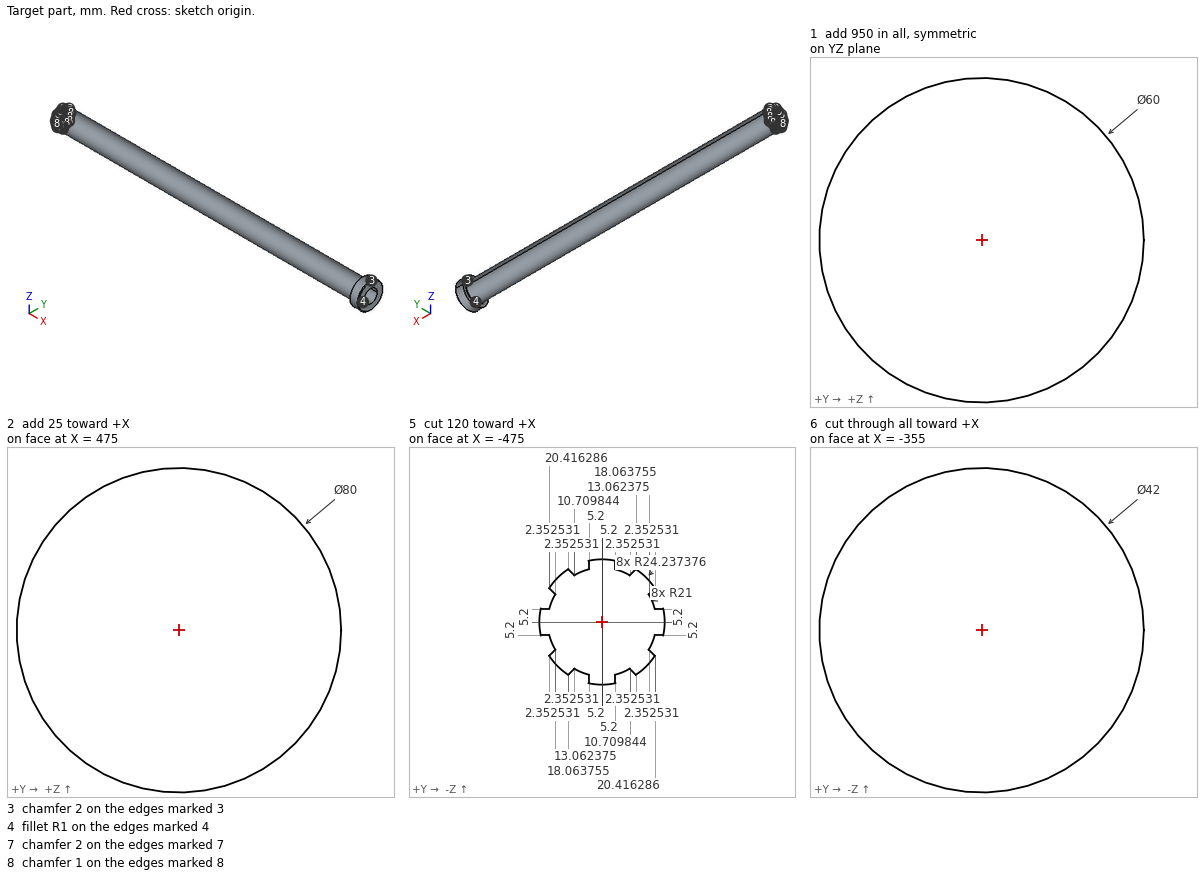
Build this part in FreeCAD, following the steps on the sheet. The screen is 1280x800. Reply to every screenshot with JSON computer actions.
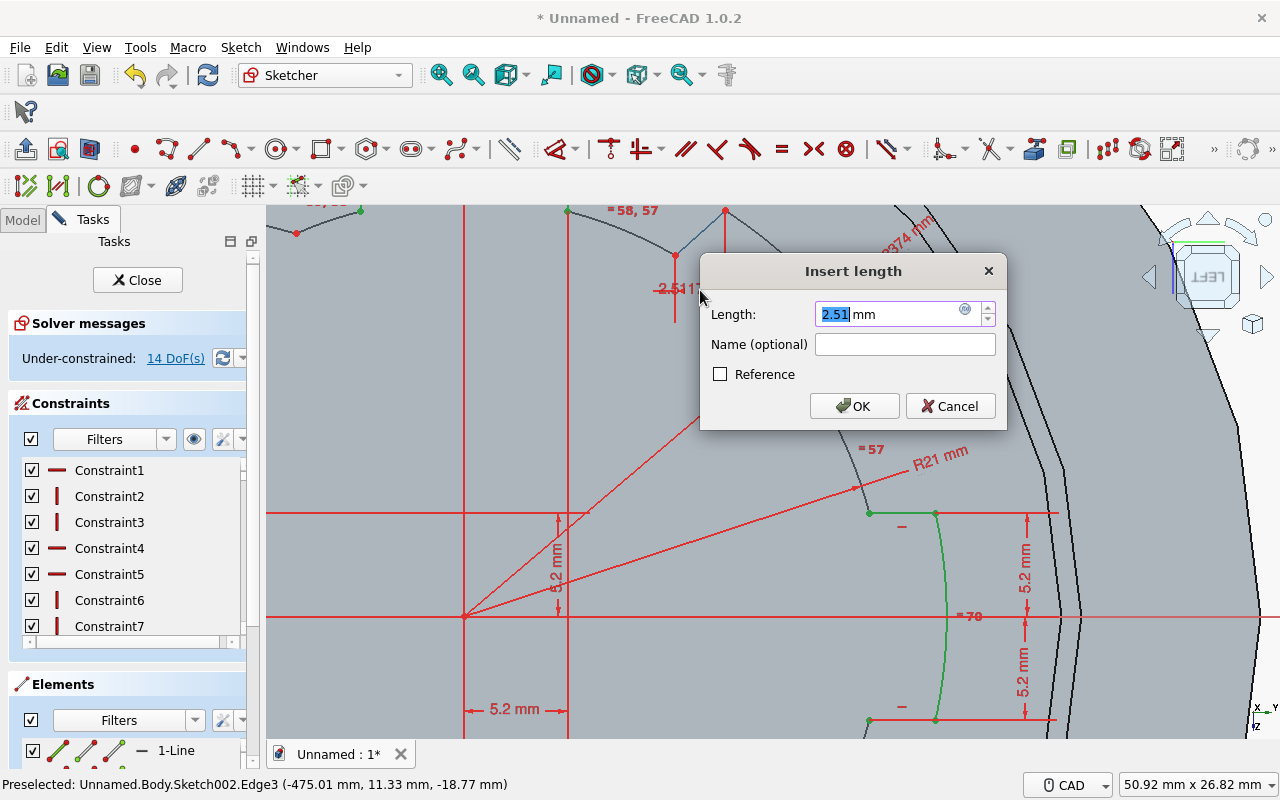
{"action": "type", "text": "2.352531"}
{"action": "key", "text": "Return"}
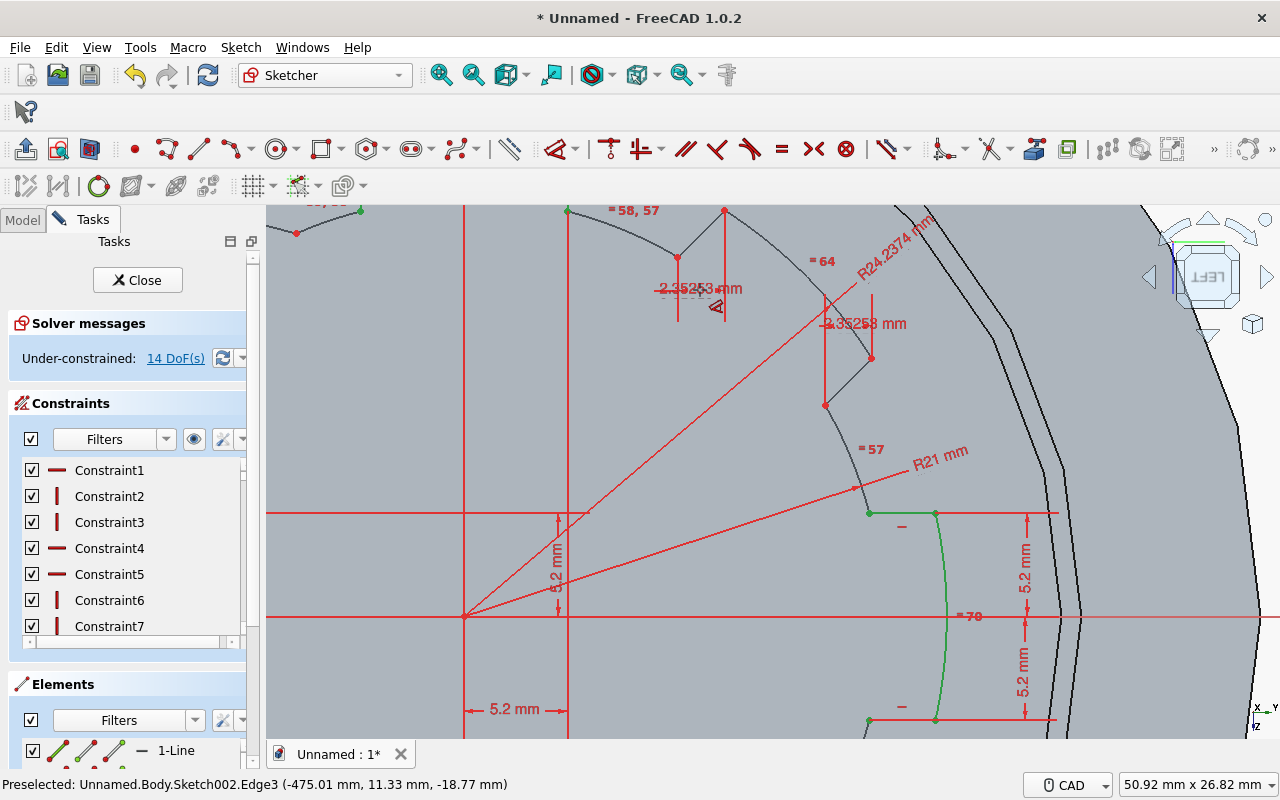
{"action": "scroll", "coordinate": [844, 388], "scroll_direction": "down", "scroll_amount": 5}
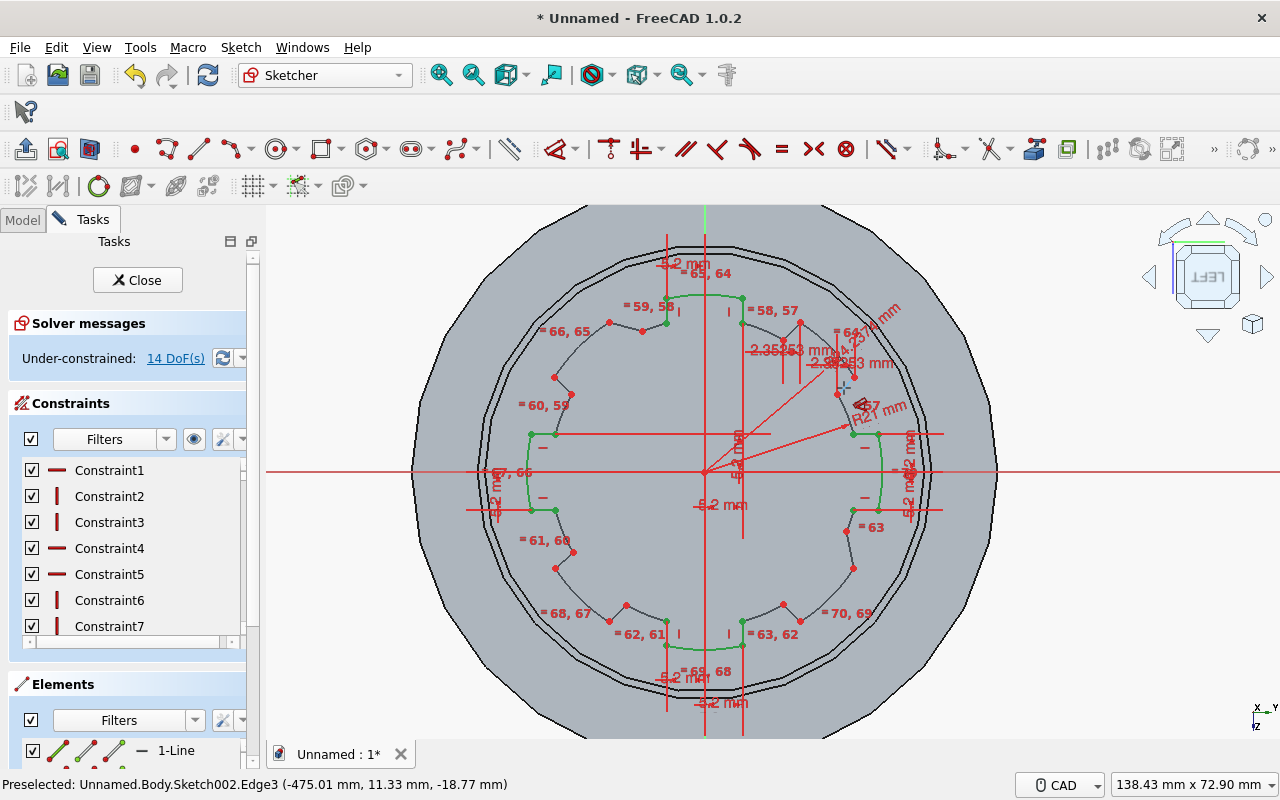
{"action": "scroll", "coordinate": [633, 329], "scroll_direction": "up", "scroll_amount": 5}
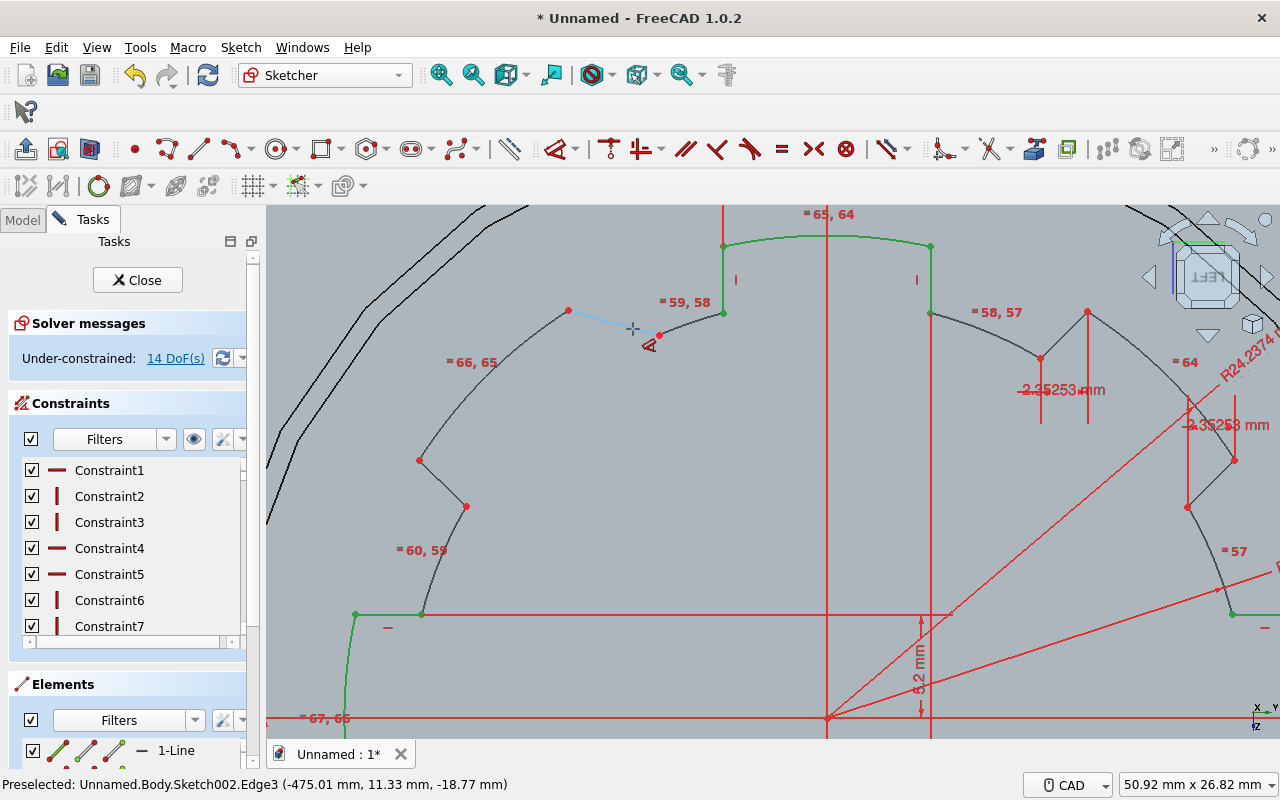
{"action": "left_click", "coordinate": [632, 328]}
{"action": "left_click", "coordinate": [614, 277]}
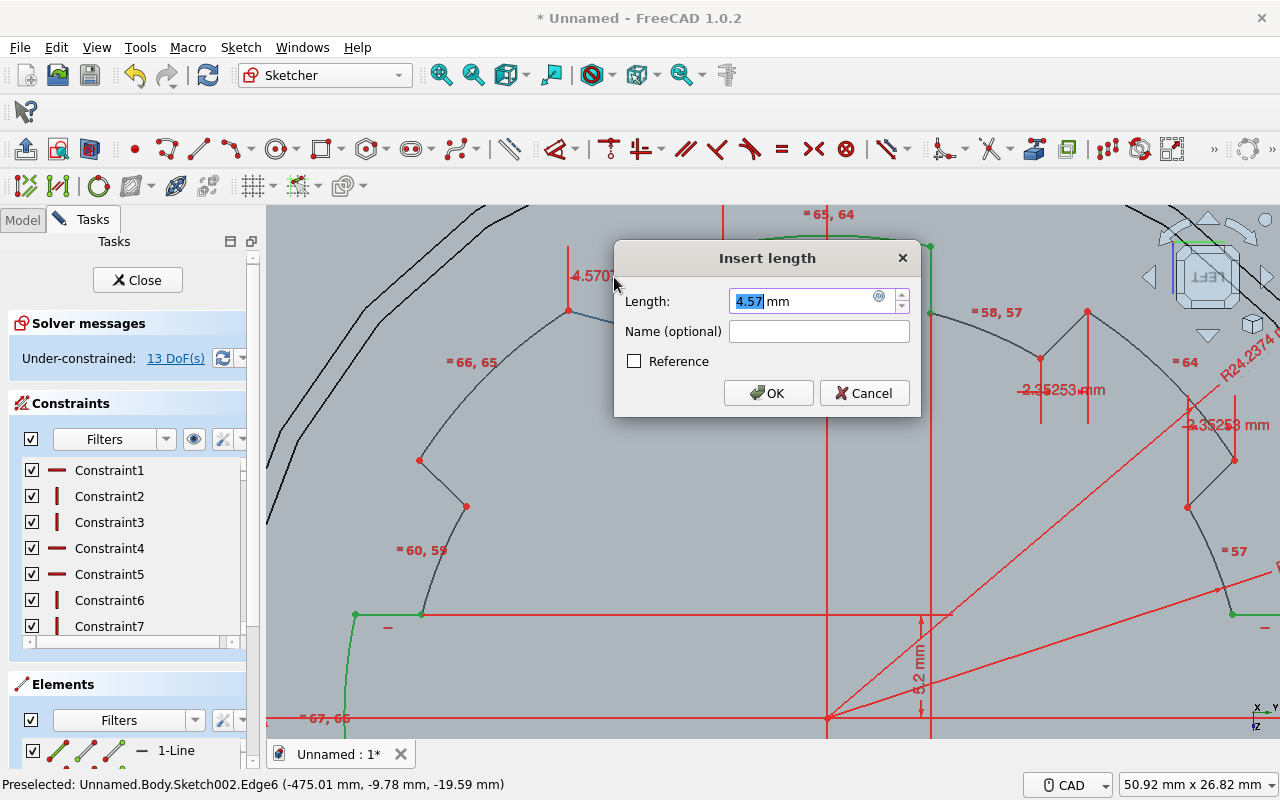
{"action": "type", "text": "2.352531"}
{"action": "key", "text": "Return"}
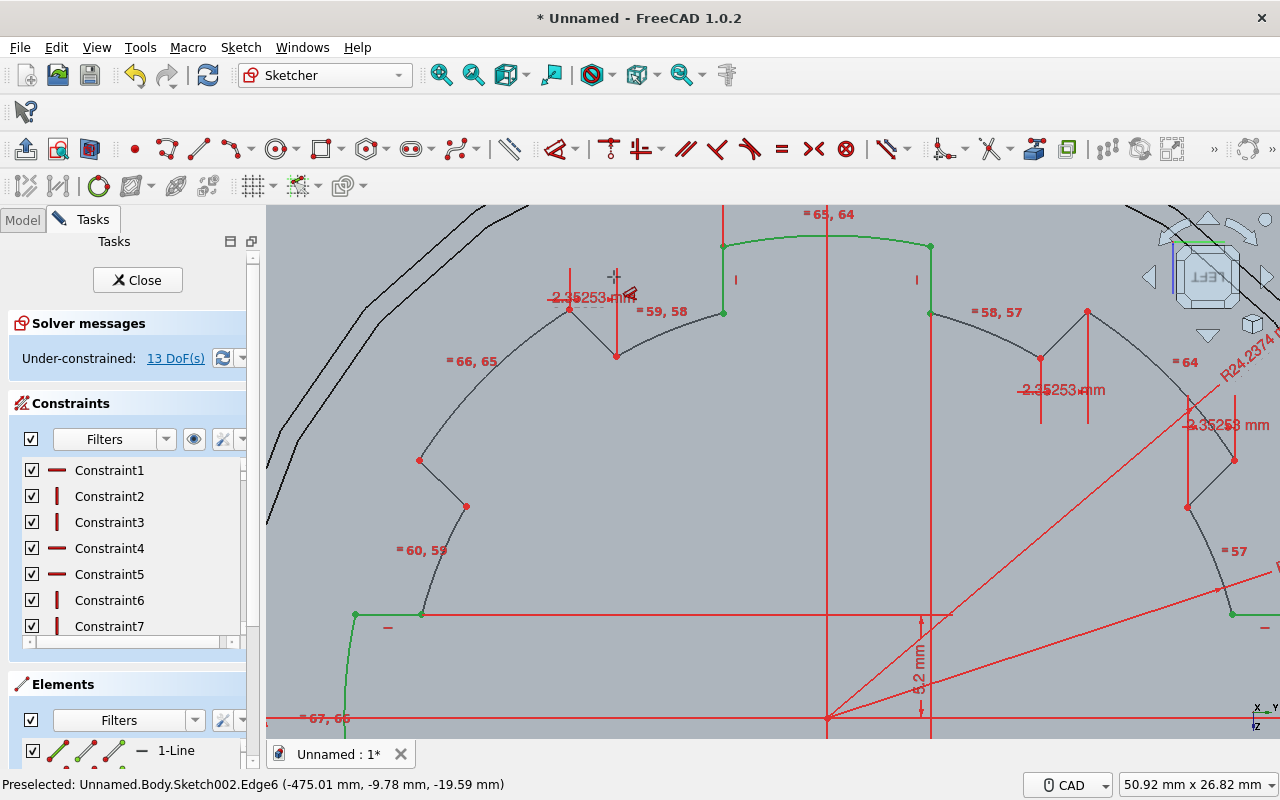
{"action": "left_click", "coordinate": [433, 474]}
{"action": "left_click", "coordinate": [426, 426]}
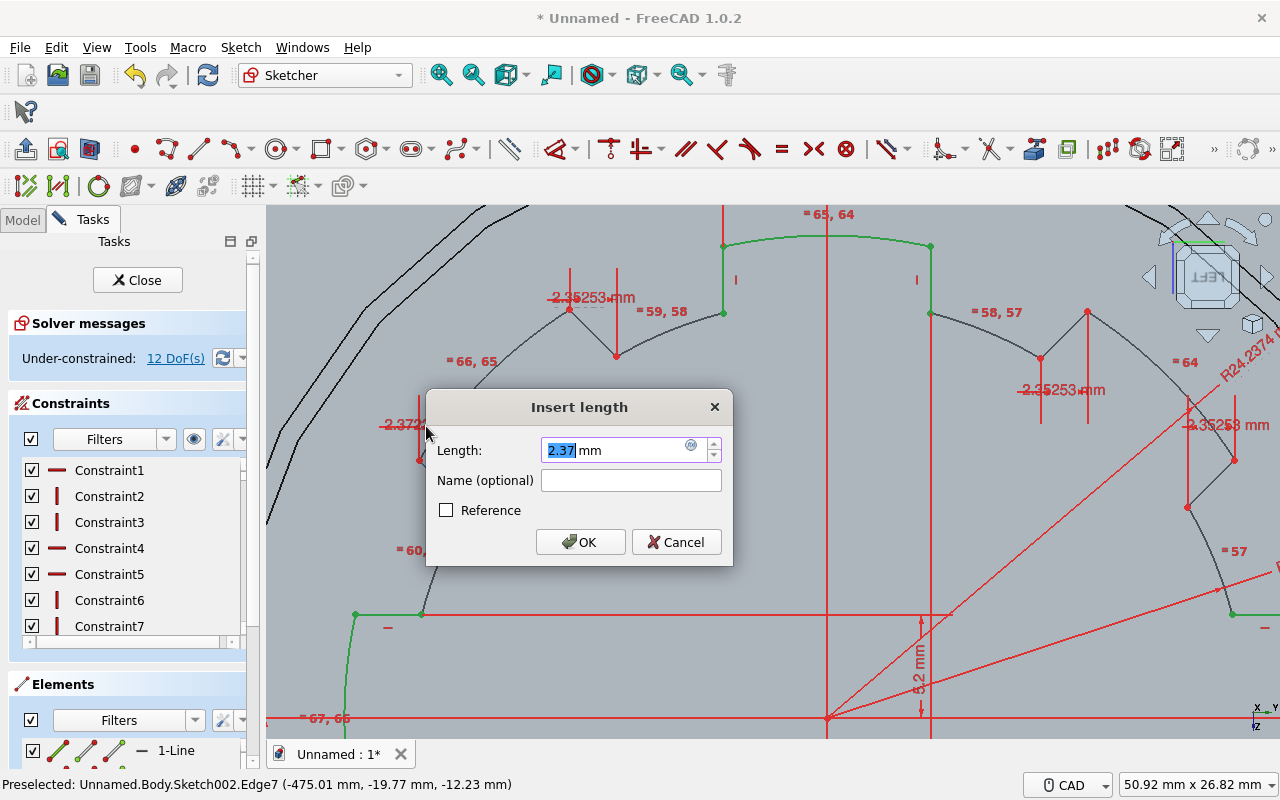
{"action": "type", "text": "2.352531"}
{"action": "key", "text": "Return"}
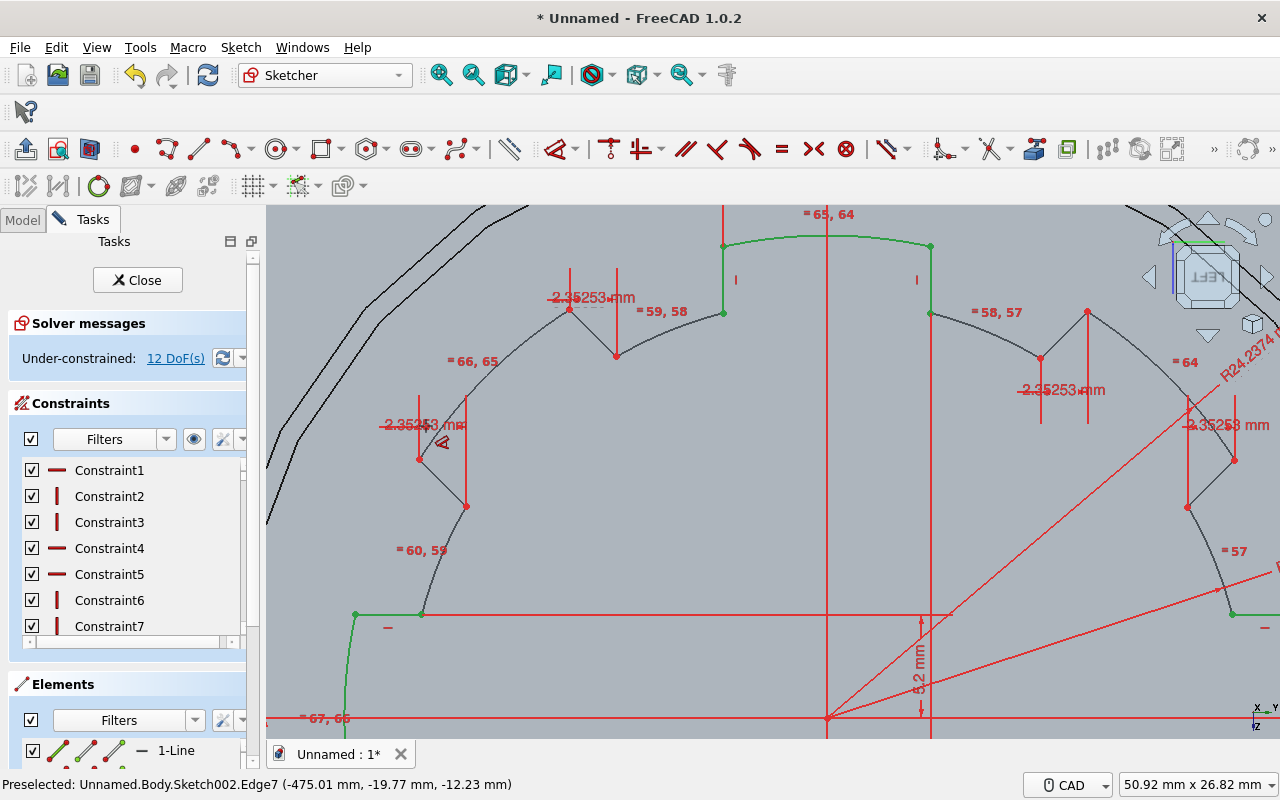
{"action": "scroll", "coordinate": [633, 329], "scroll_direction": "down", "scroll_amount": 5}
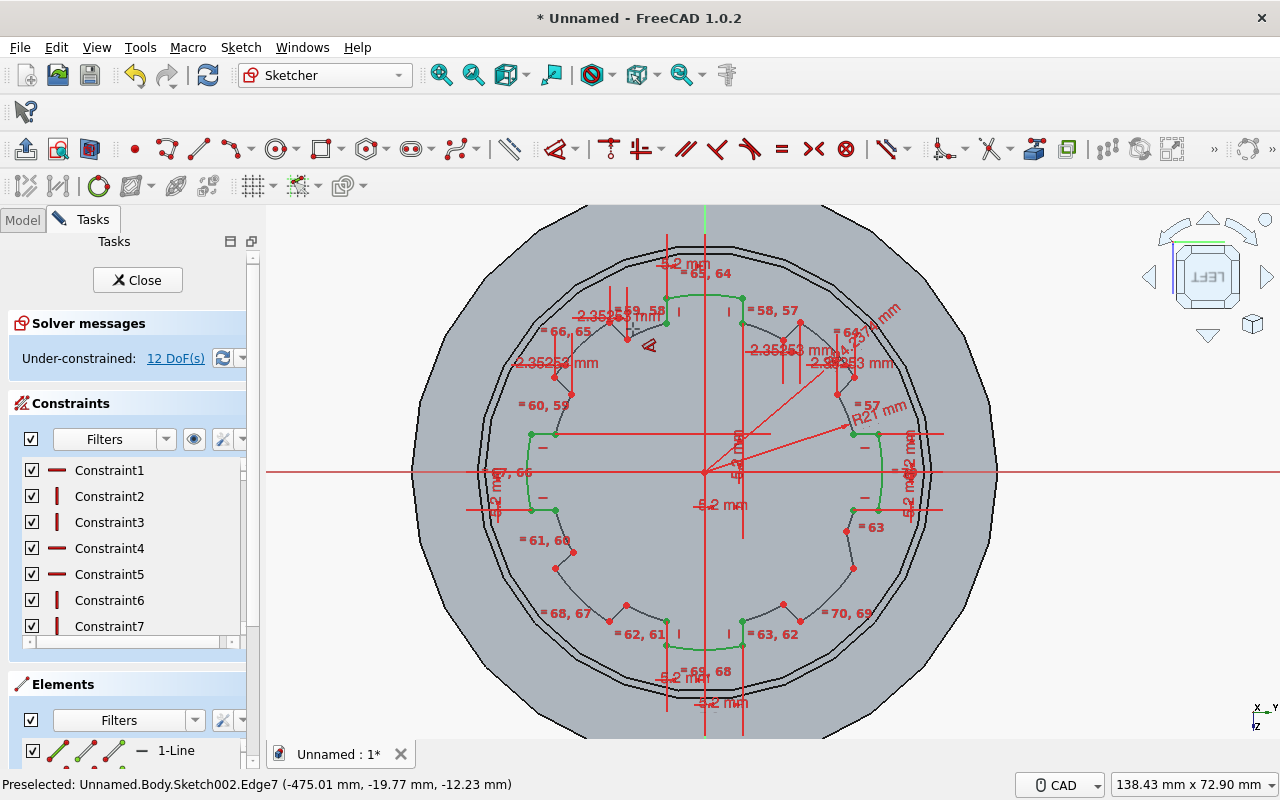
{"action": "scroll", "coordinate": [568, 557], "scroll_direction": "up", "scroll_amount": 5}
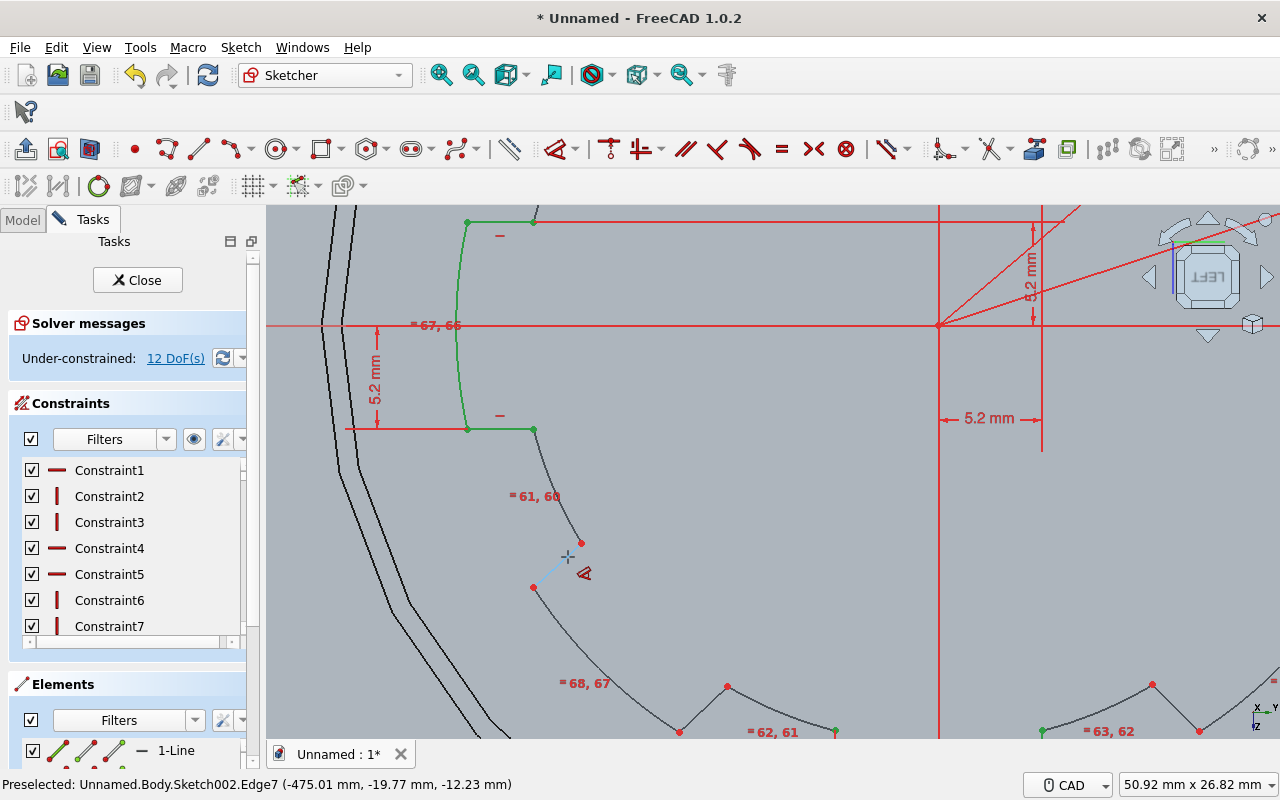
{"action": "left_click", "coordinate": [567, 557]}
{"action": "left_click", "coordinate": [541, 622]}